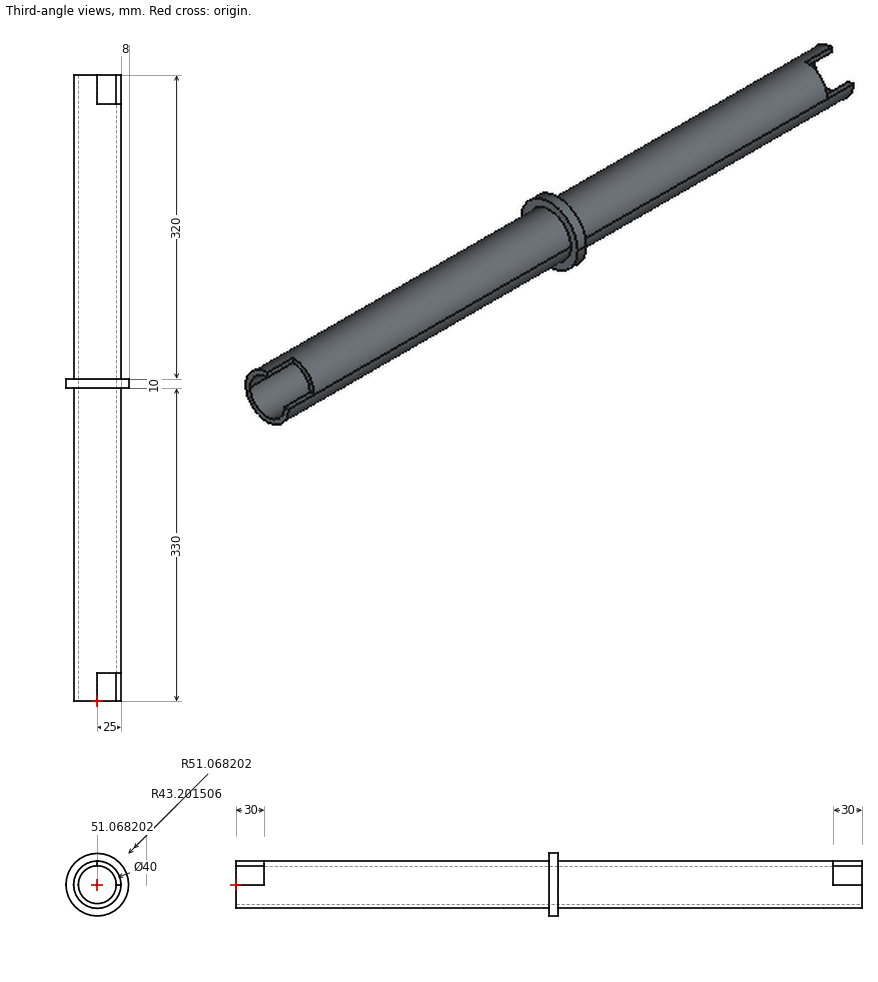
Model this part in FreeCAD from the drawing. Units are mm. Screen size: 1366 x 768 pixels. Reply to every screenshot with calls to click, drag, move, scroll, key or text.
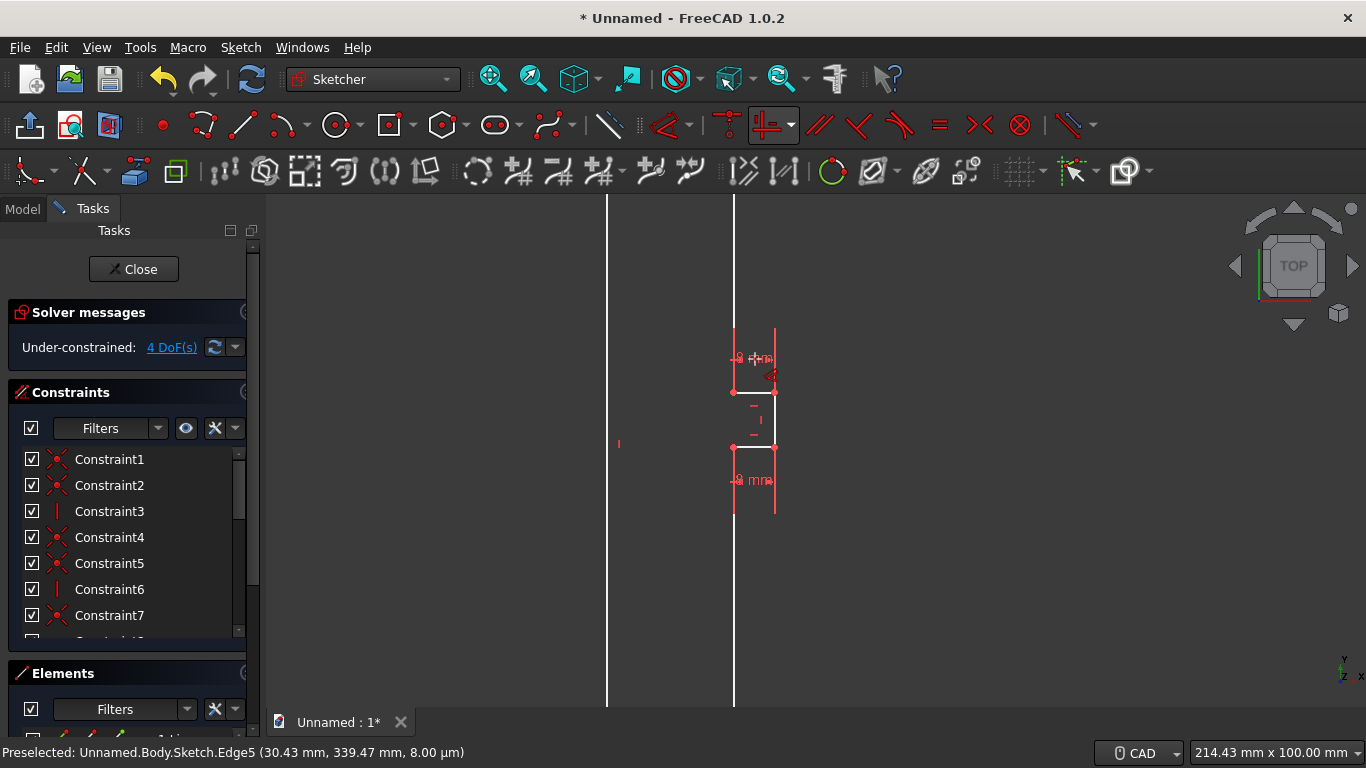
scroll(753, 451, down, 12)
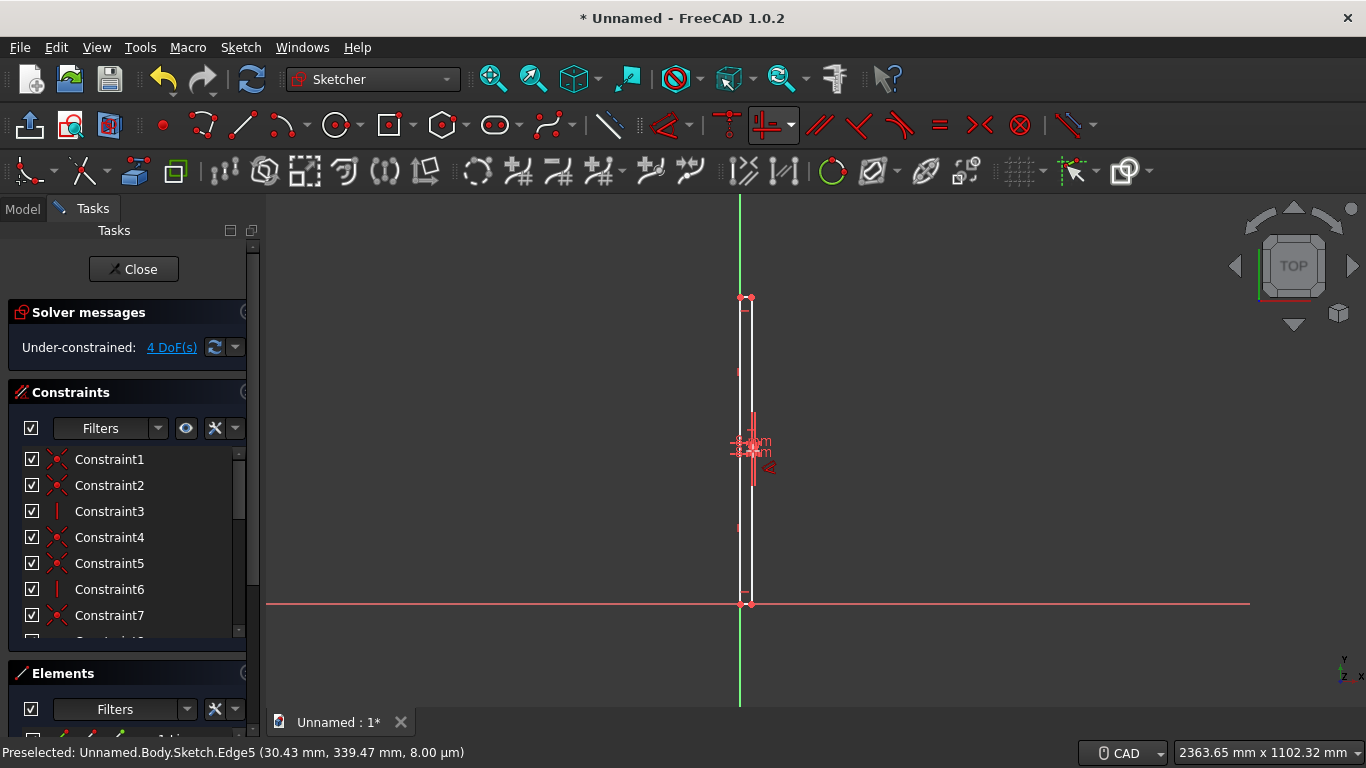
scroll(744, 604, up, 7)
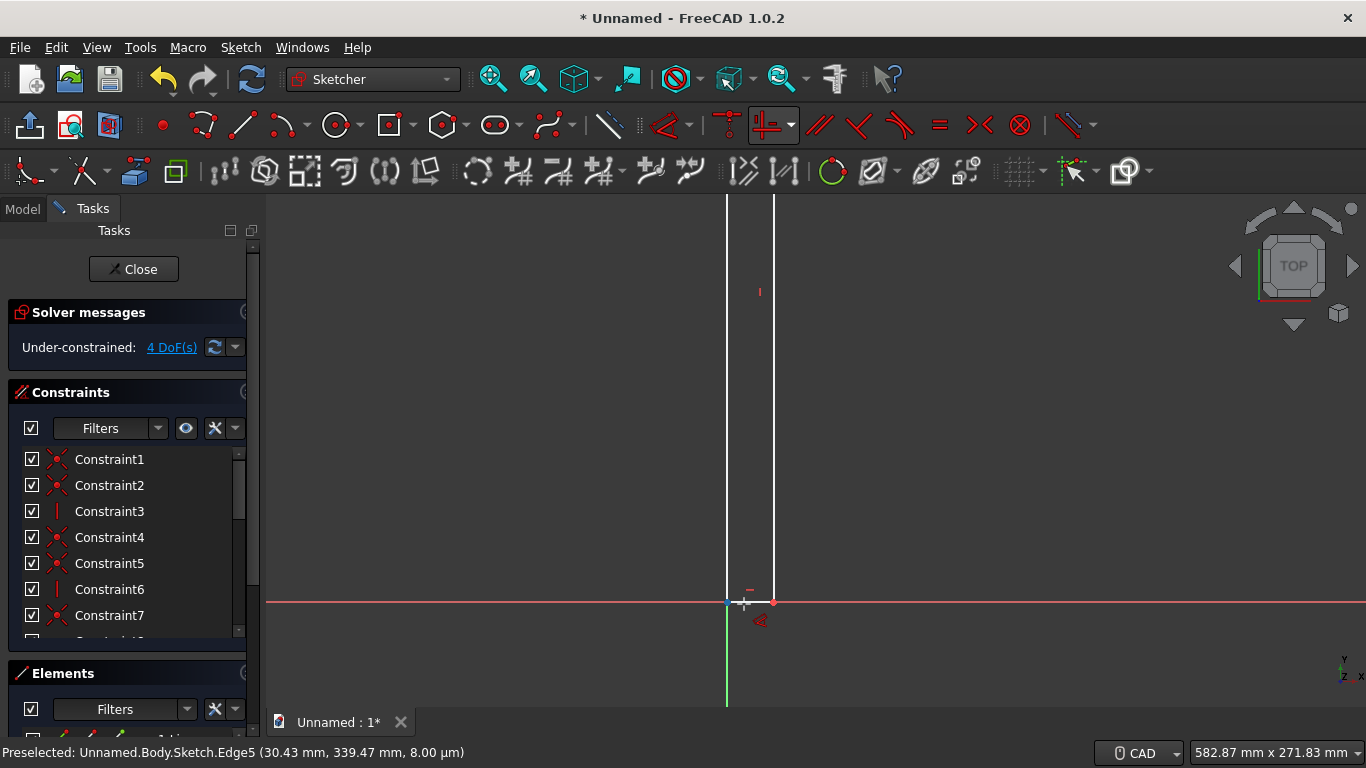
click(741, 602)
click(750, 636)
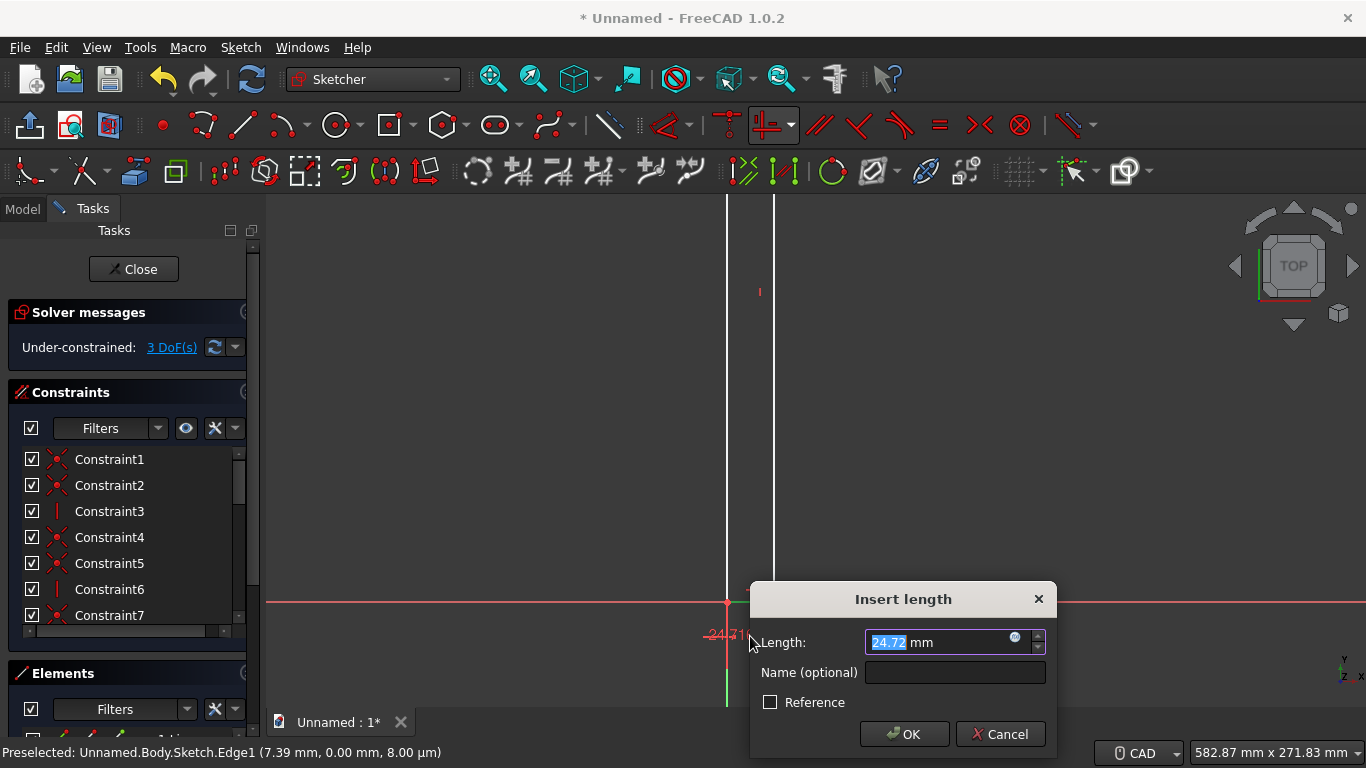
text(25)
key(Return)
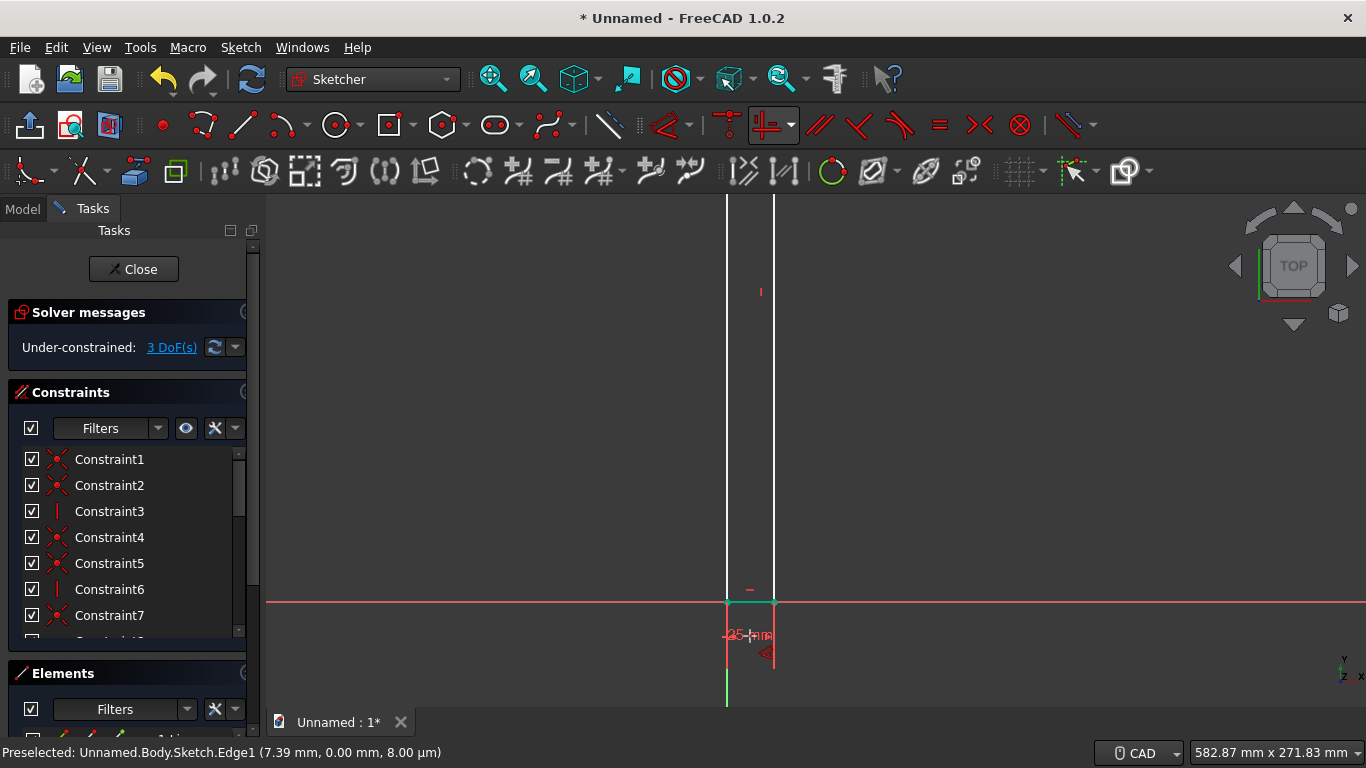
scroll(744, 605, down, 7)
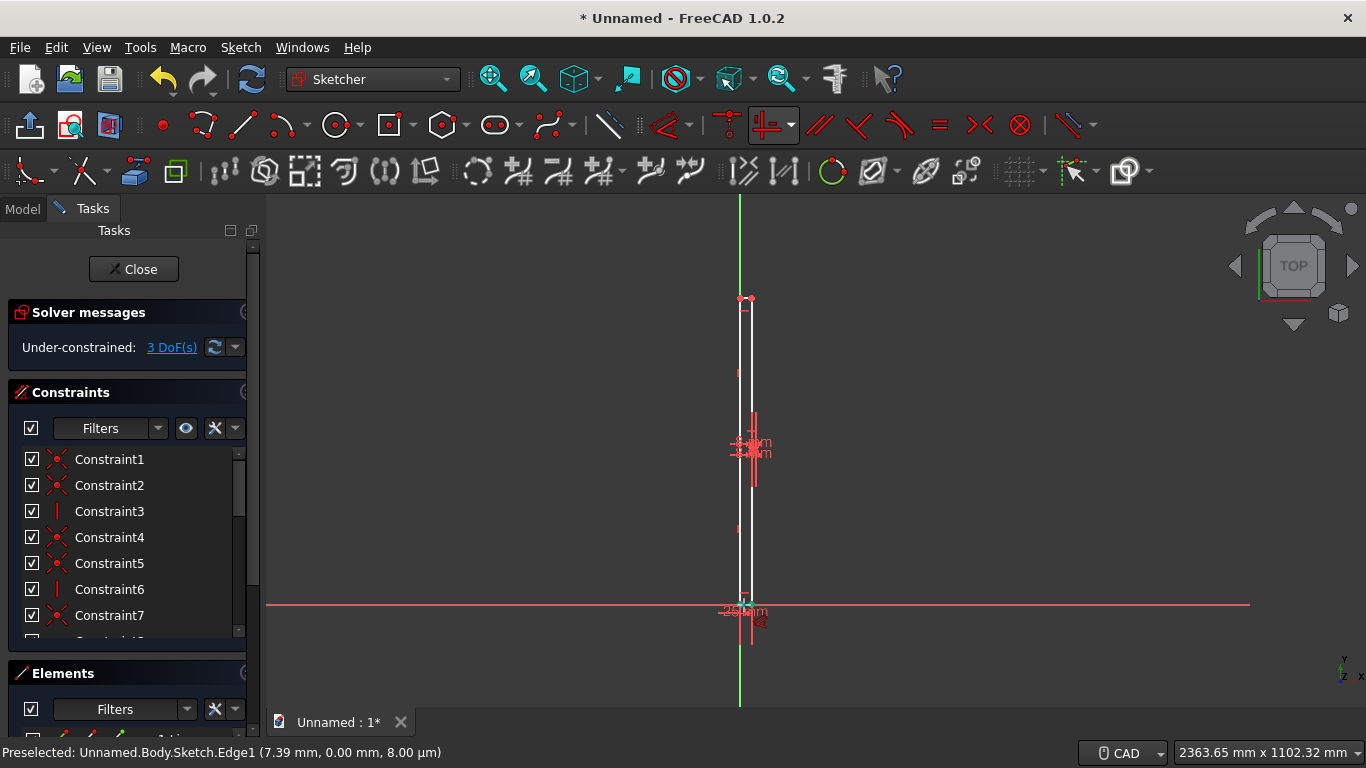
scroll(756, 449, up, 11)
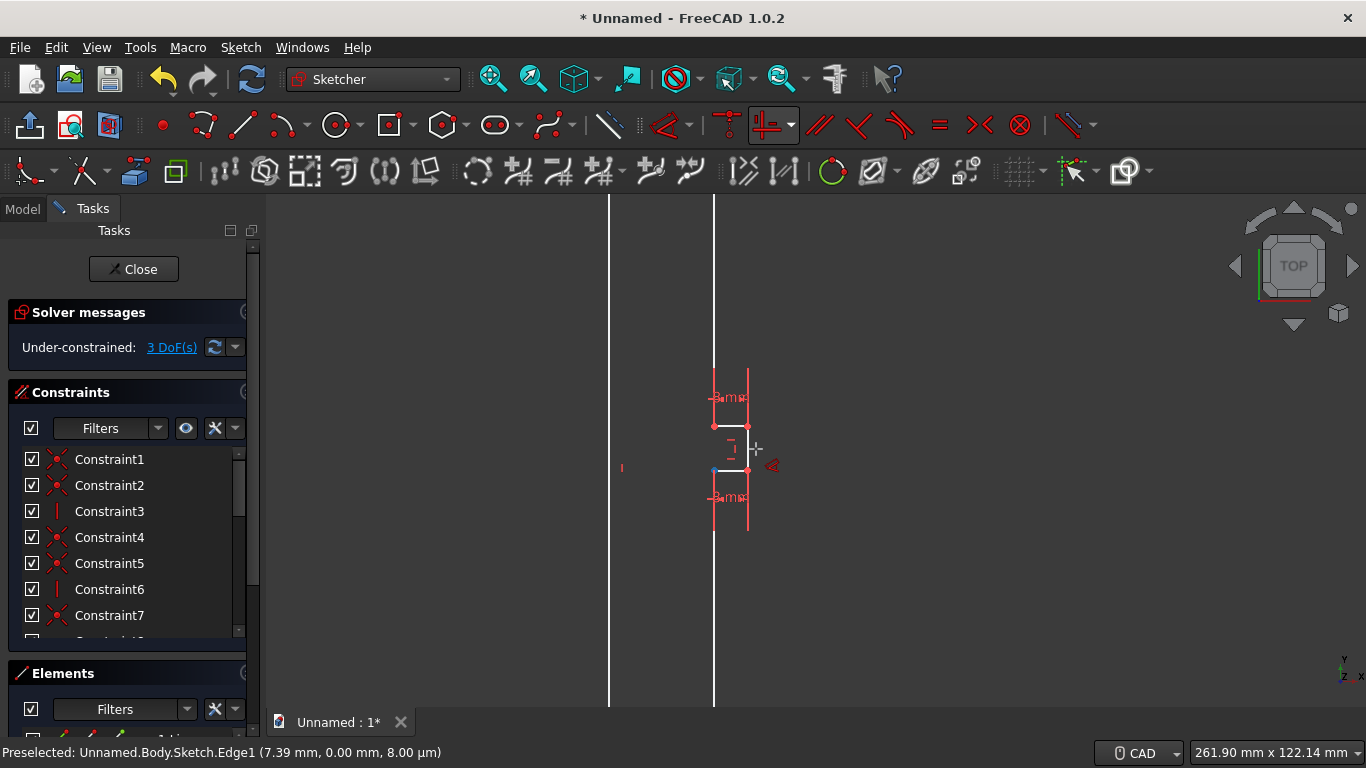
click(748, 449)
click(782, 449)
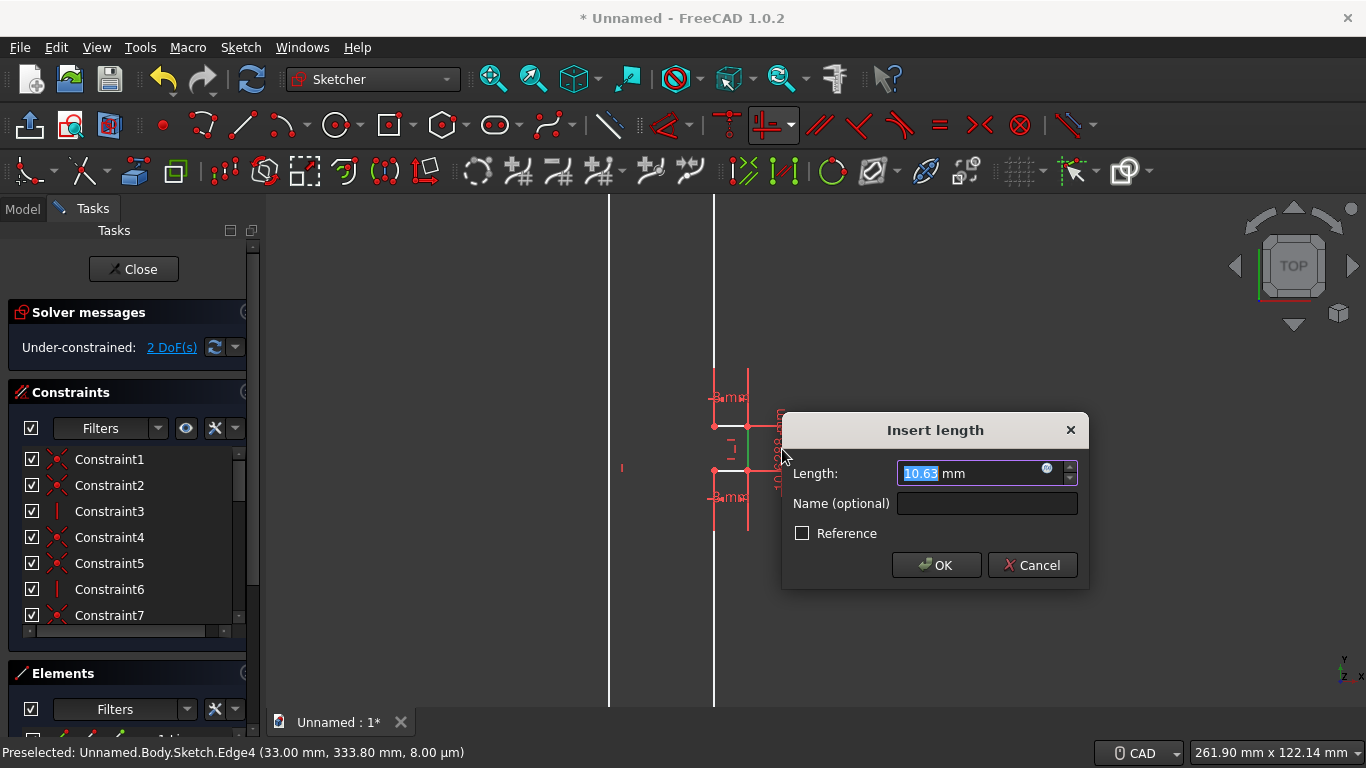
text(10)
key(Return)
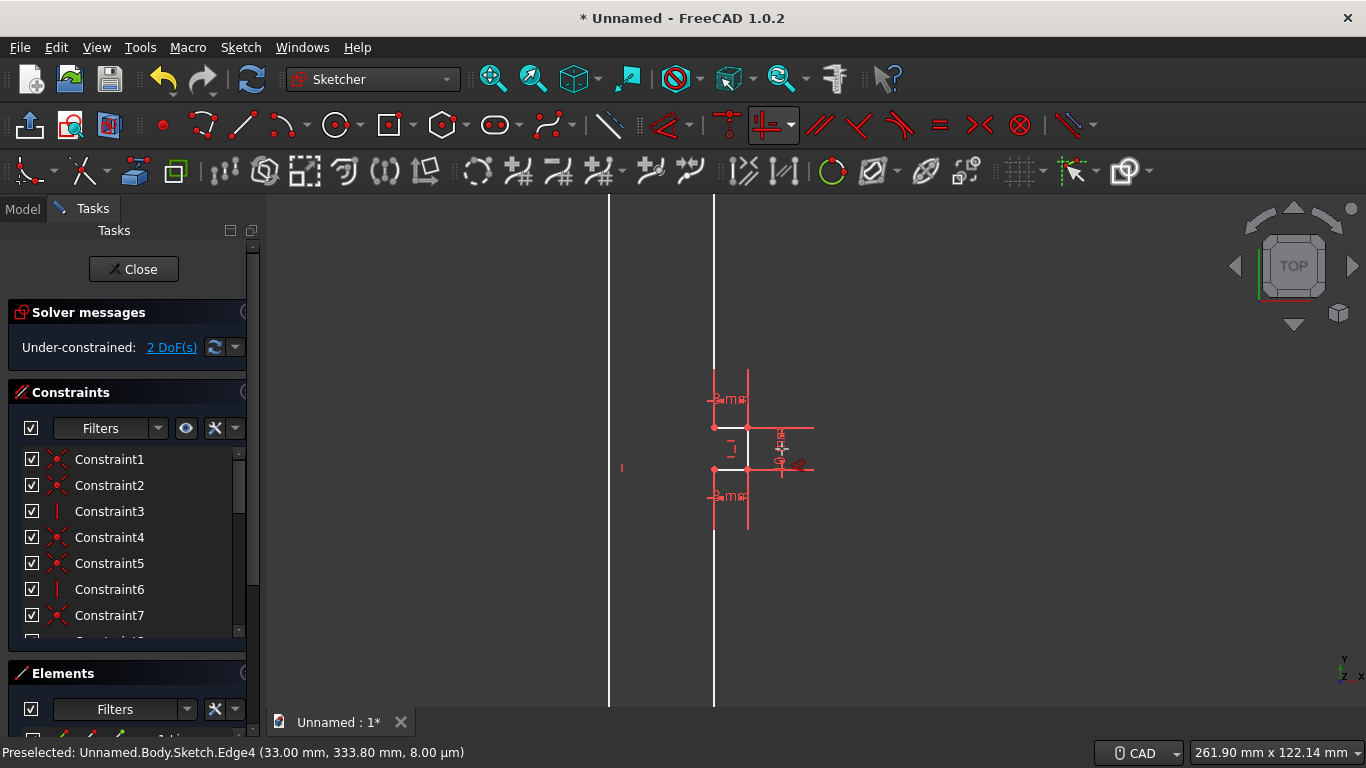
scroll(756, 449, down, 11)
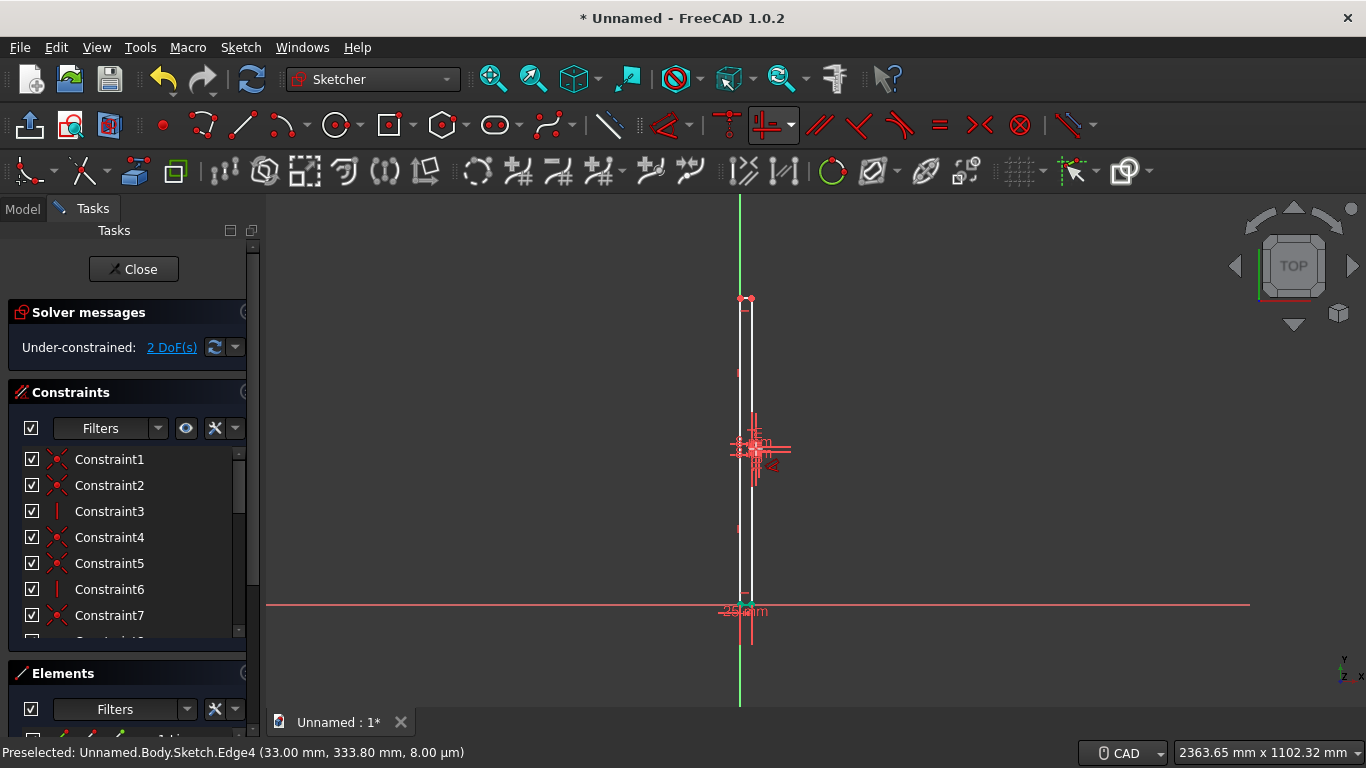
click(752, 559)
click(786, 528)